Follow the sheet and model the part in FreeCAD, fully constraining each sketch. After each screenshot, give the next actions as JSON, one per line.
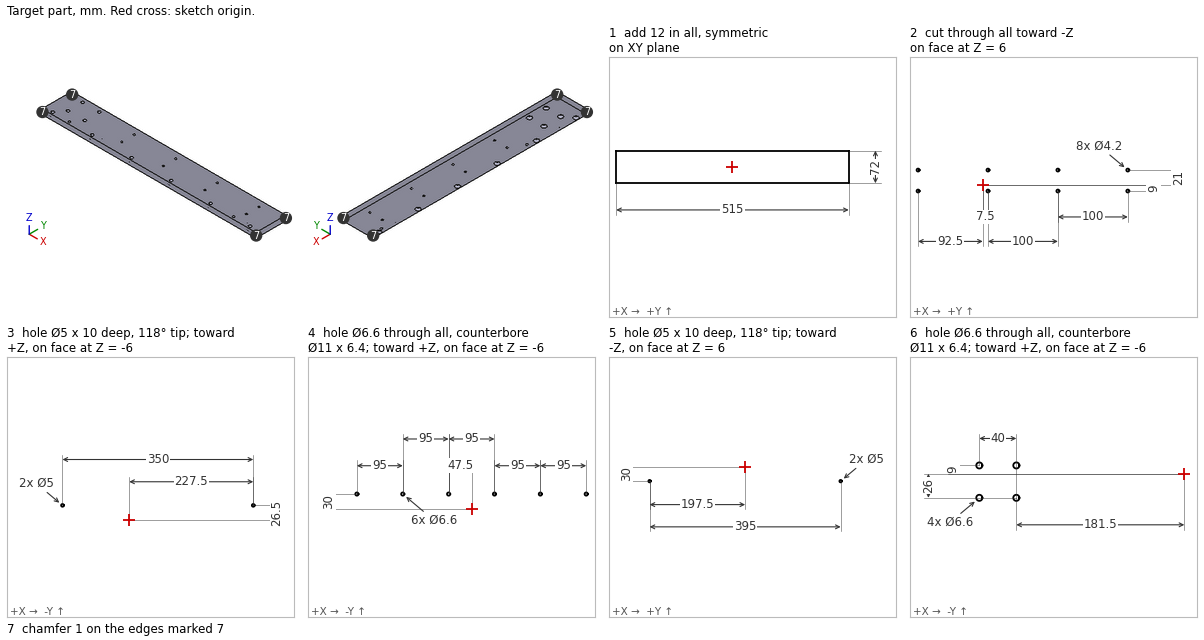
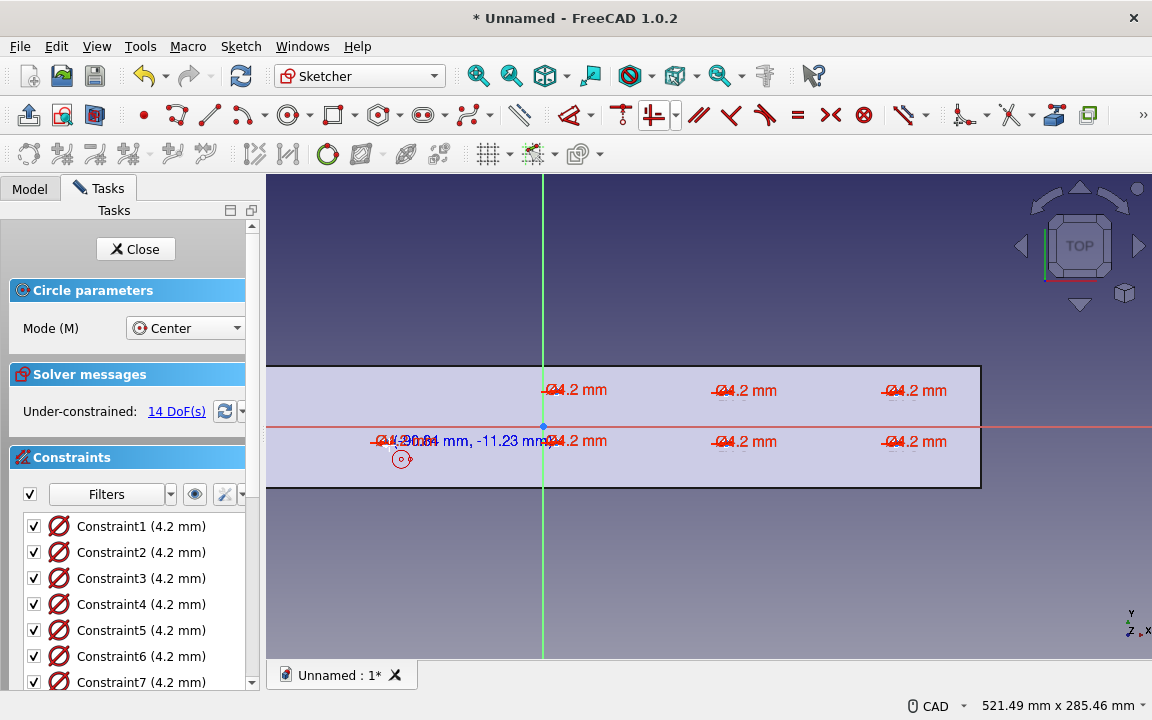
{"action": "scroll", "coordinate": [386, 391], "scroll_direction": "up", "scroll_amount": 10}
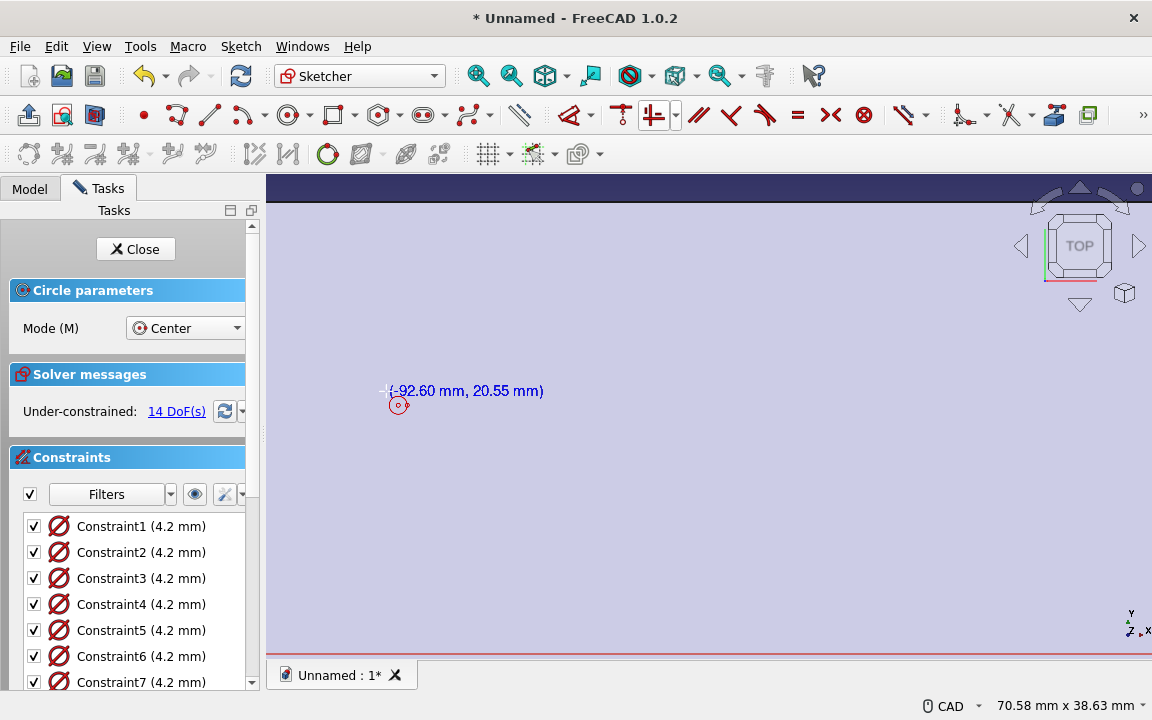
{"action": "scroll", "coordinate": [386, 391], "scroll_direction": "down", "scroll_amount": 10}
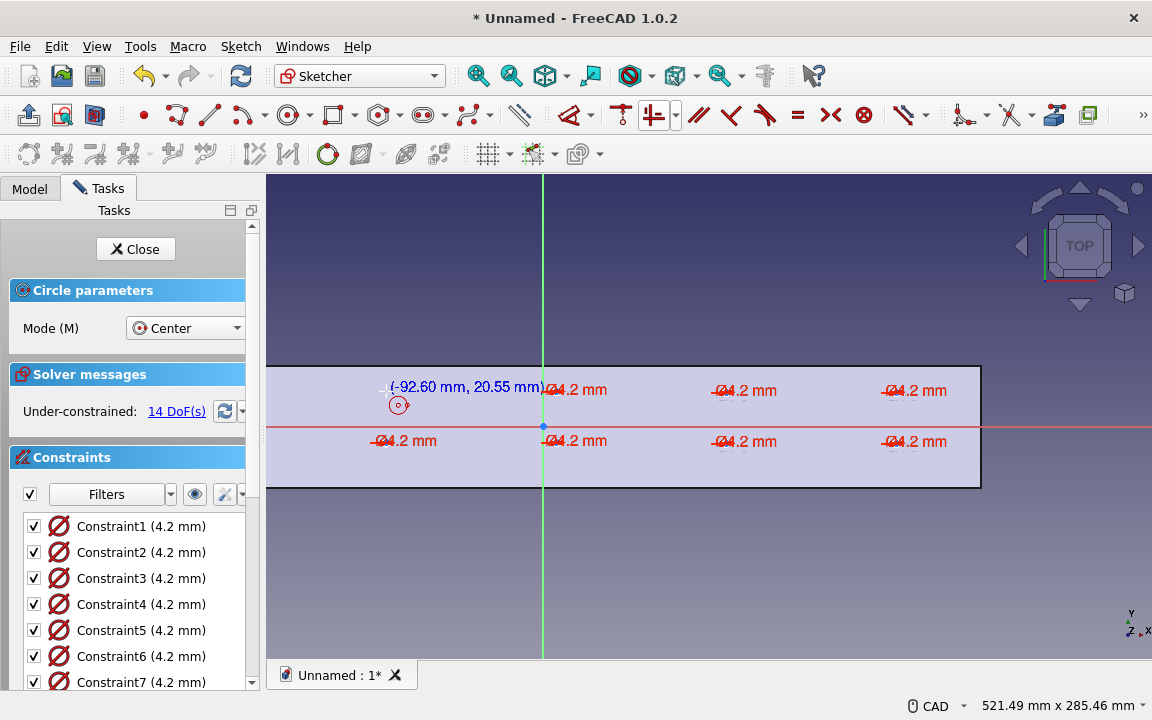
{"action": "left_click", "coordinate": [386, 391]}
{"action": "mouse_move", "coordinate": [389, 389]}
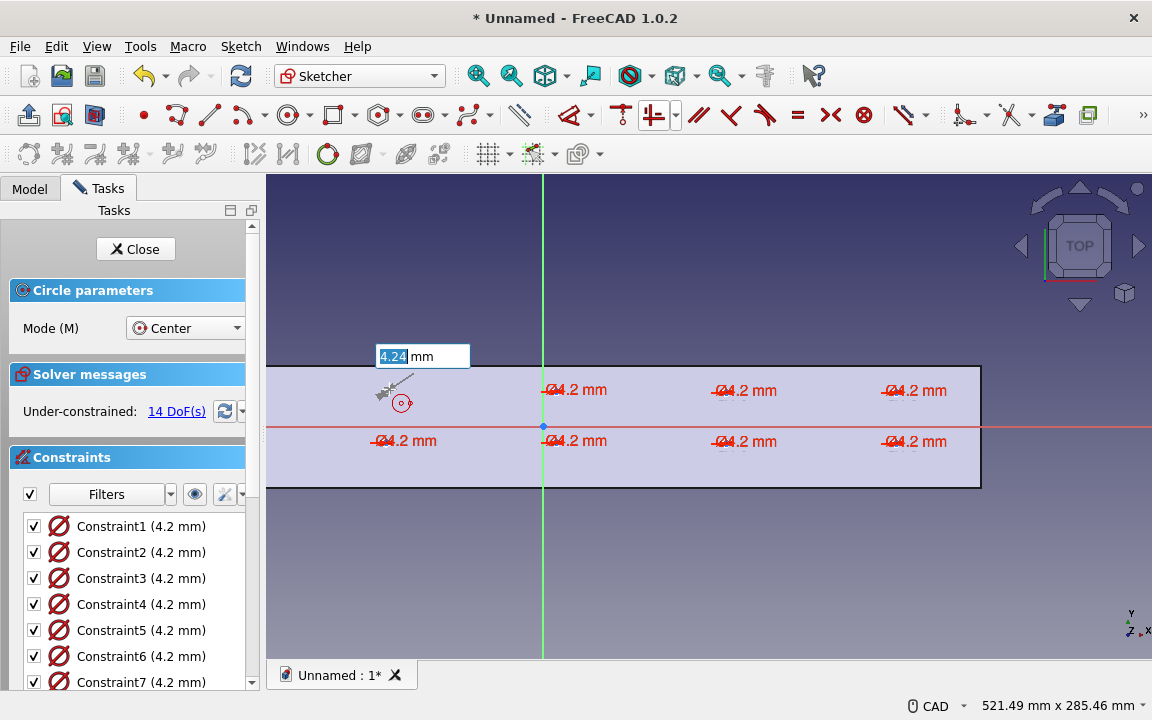
{"action": "type", "text": "4.2"}
{"action": "key", "text": "Return"}
{"action": "key", "text": "Escape"}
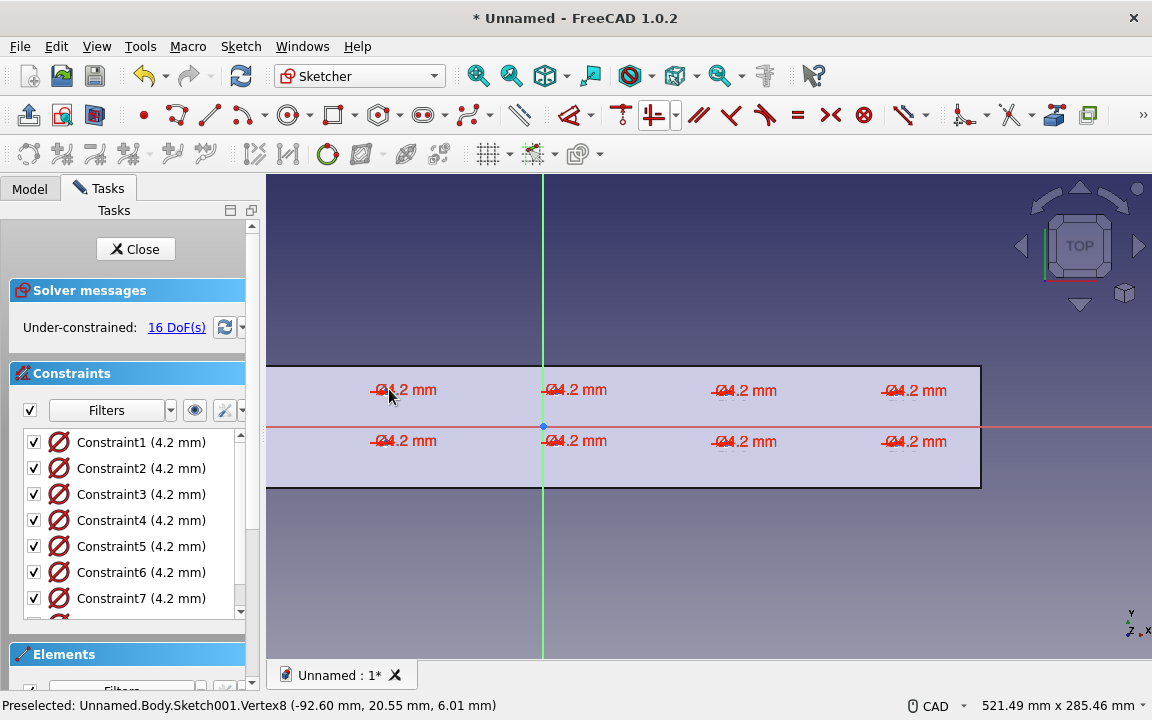
{"action": "left_click", "coordinate": [896, 444]}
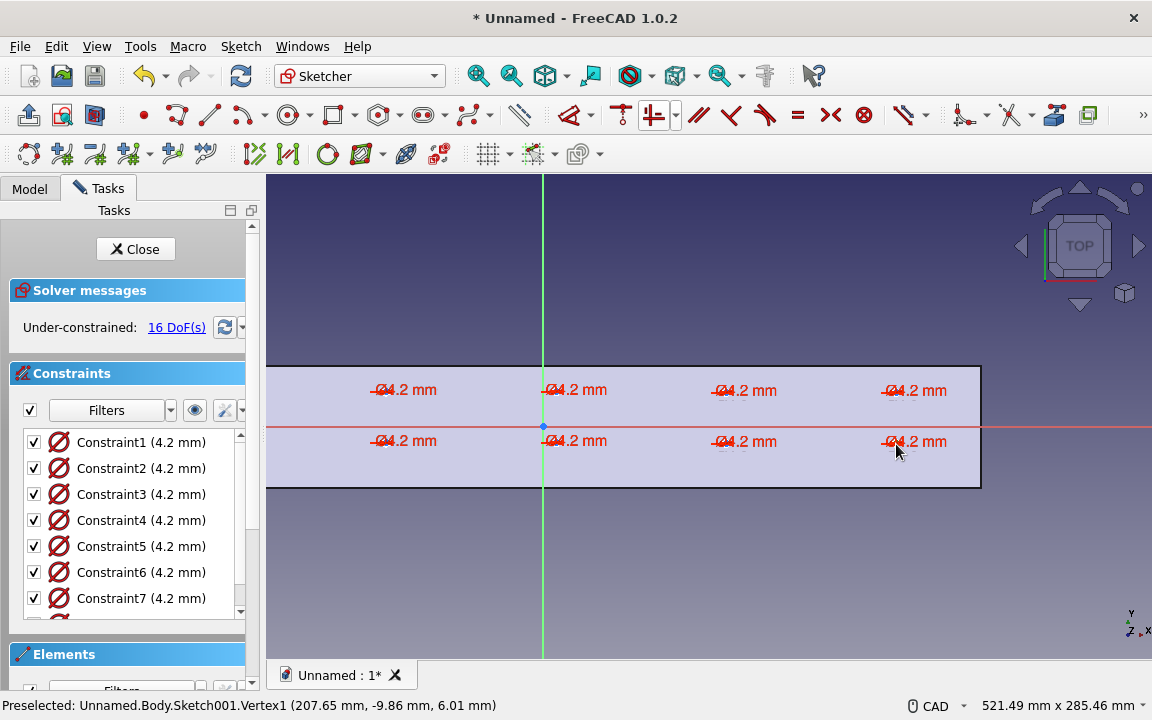
{"action": "left_click", "coordinate": [896, 393]}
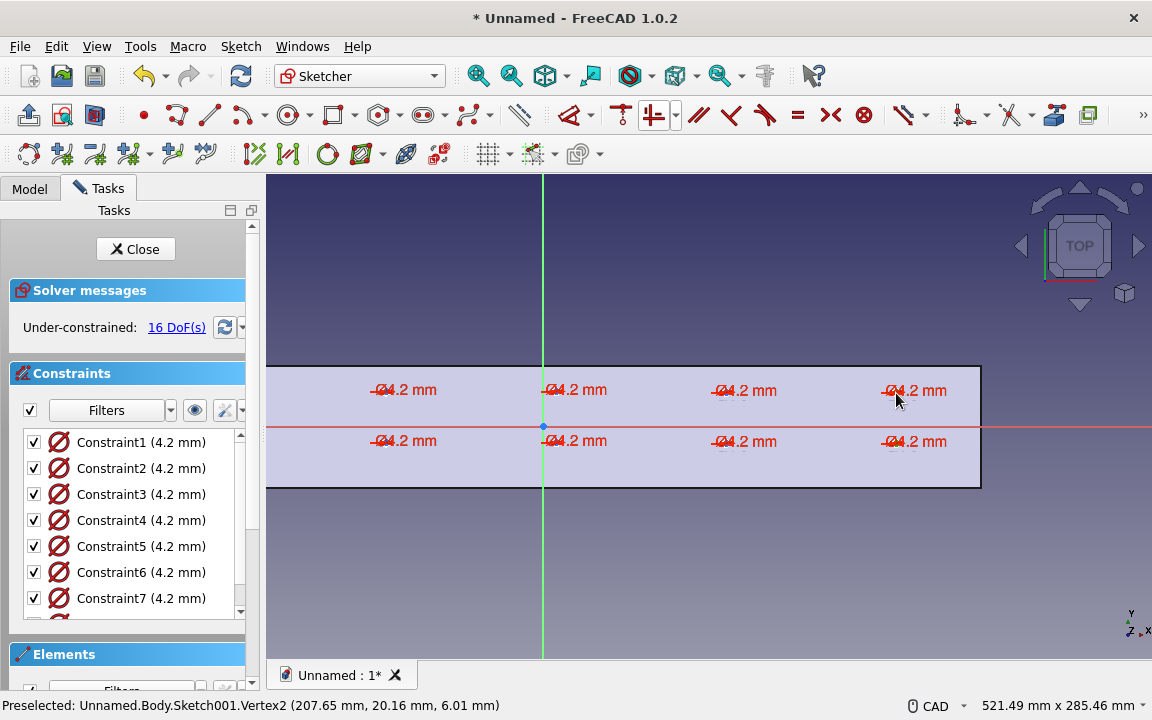
{"action": "left_click", "coordinate": [676, 116]}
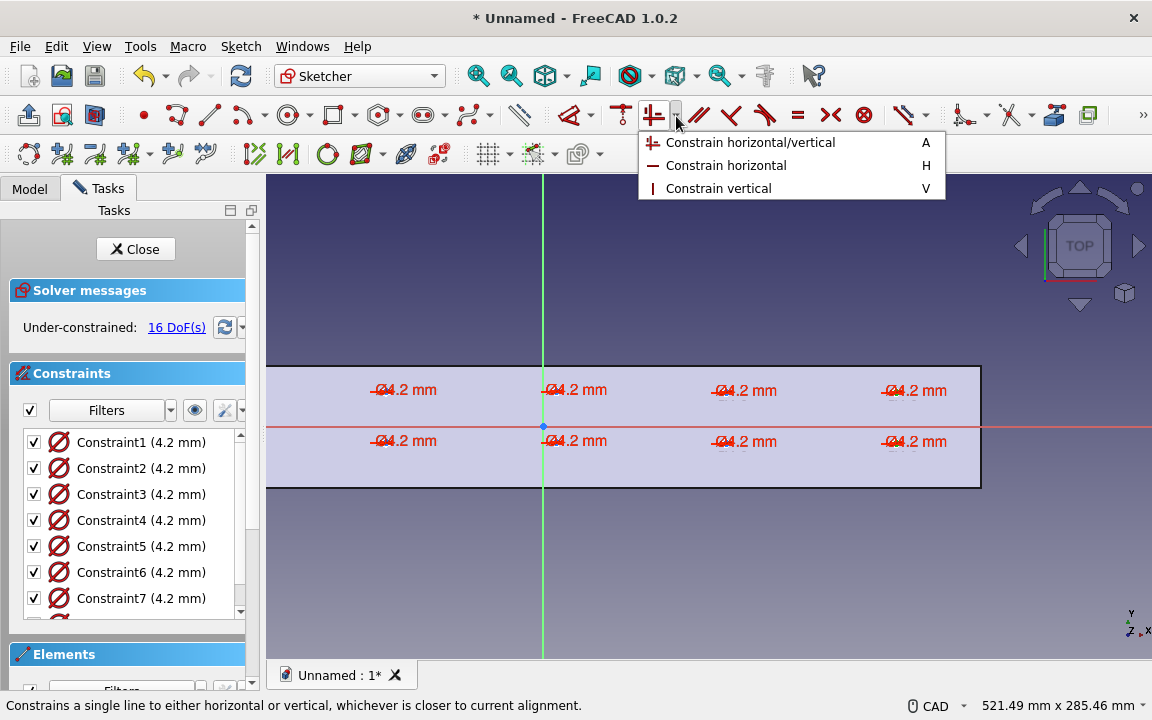
{"action": "left_click", "coordinate": [792, 188]}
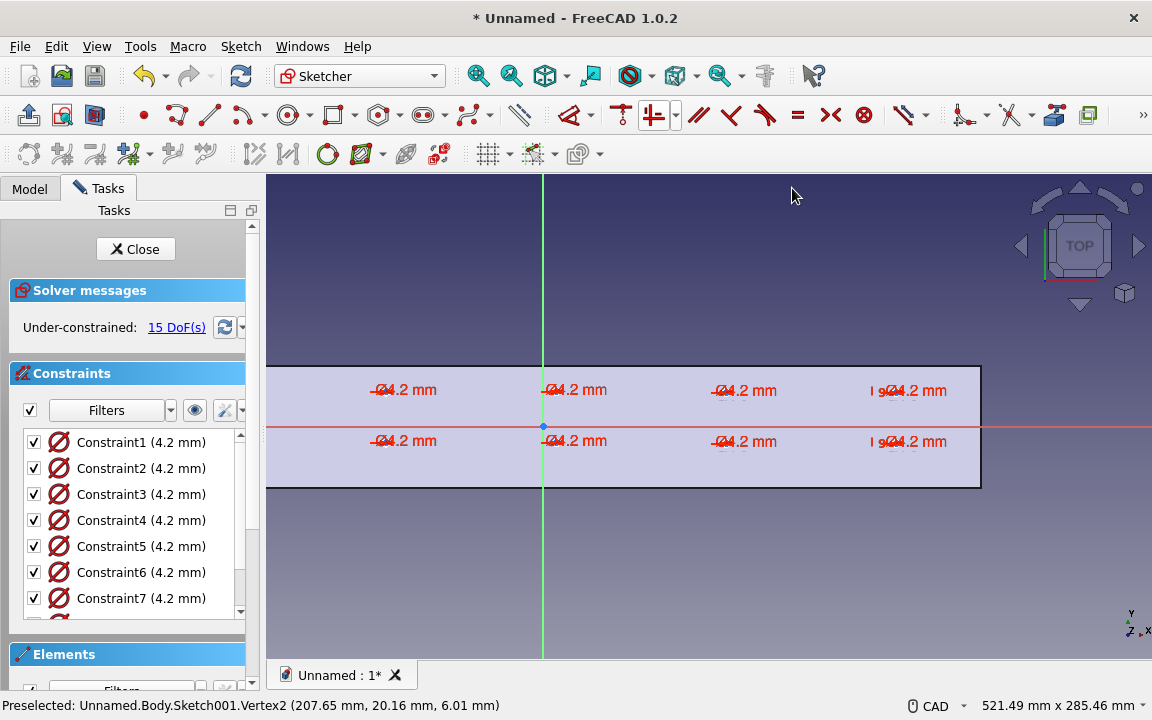
{"action": "left_click", "coordinate": [896, 444]}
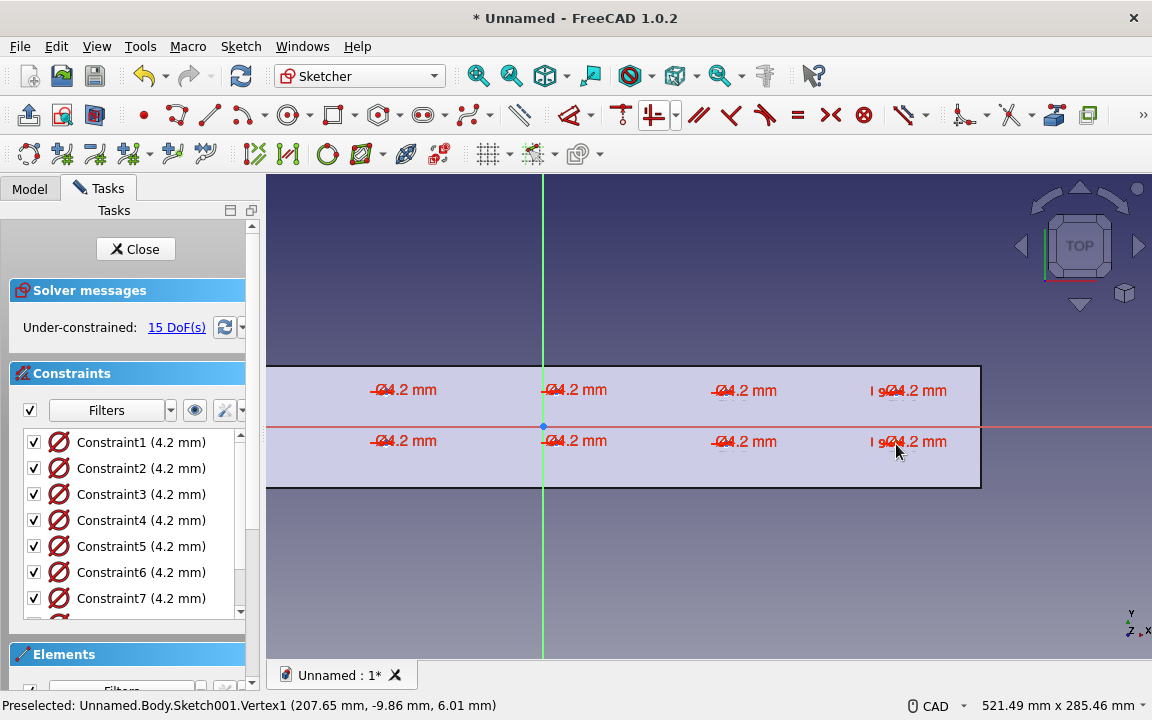
{"action": "left_click", "coordinate": [726, 444]}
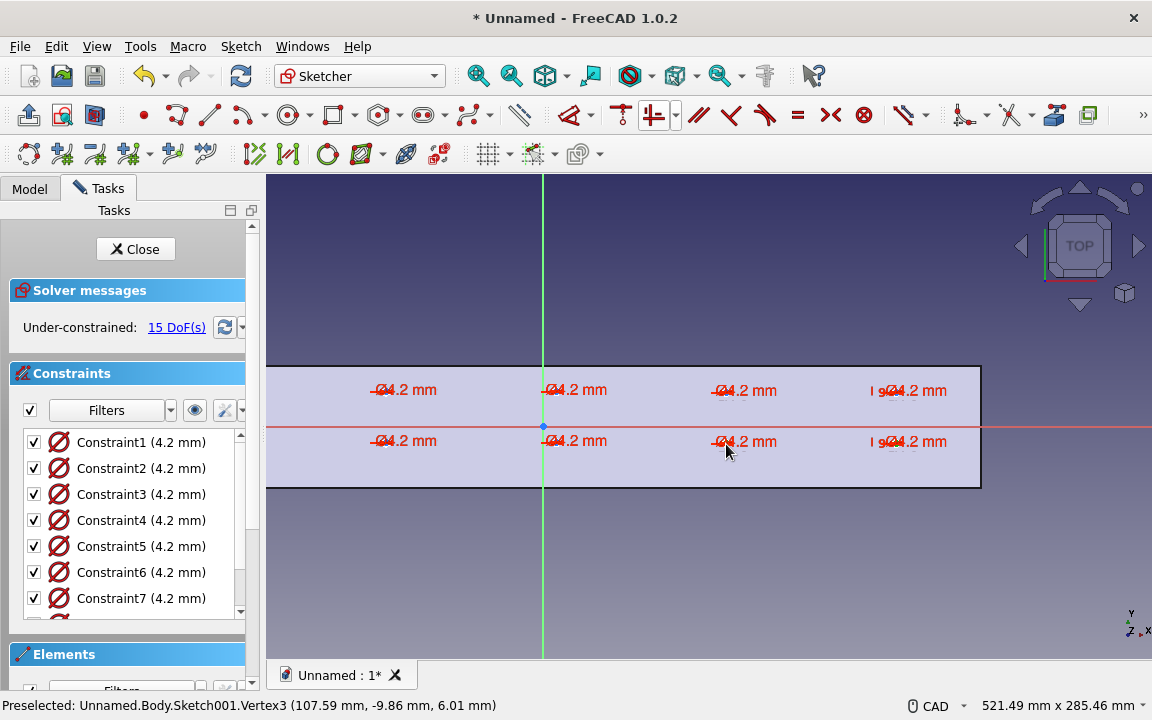
{"action": "left_click", "coordinate": [676, 116]}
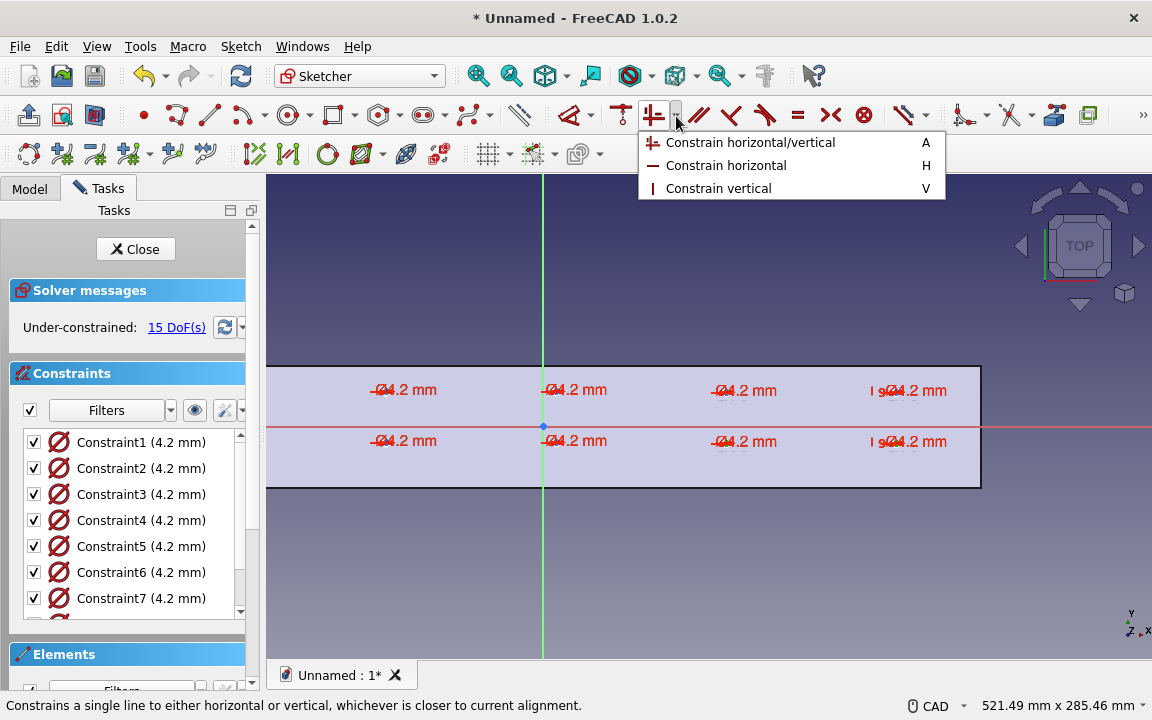
{"action": "left_click", "coordinate": [792, 166]}